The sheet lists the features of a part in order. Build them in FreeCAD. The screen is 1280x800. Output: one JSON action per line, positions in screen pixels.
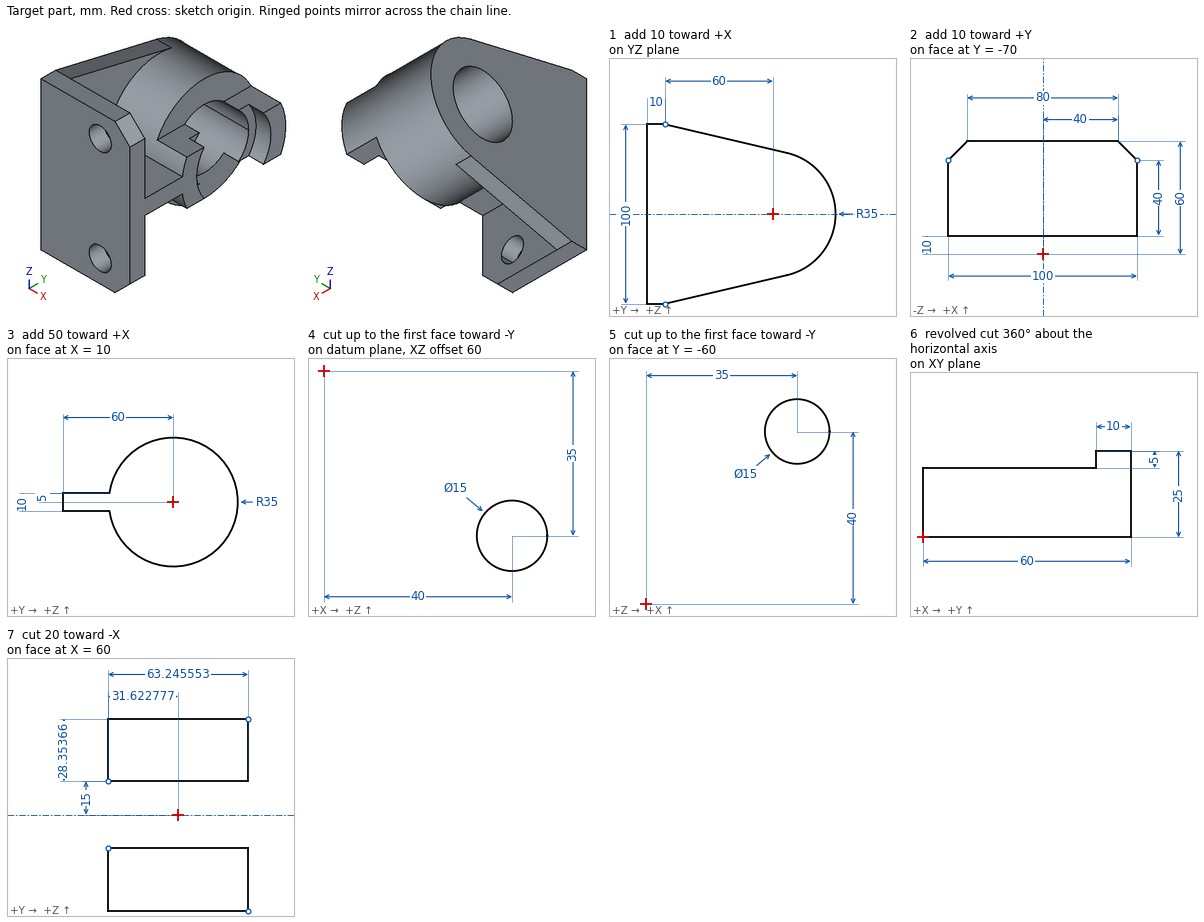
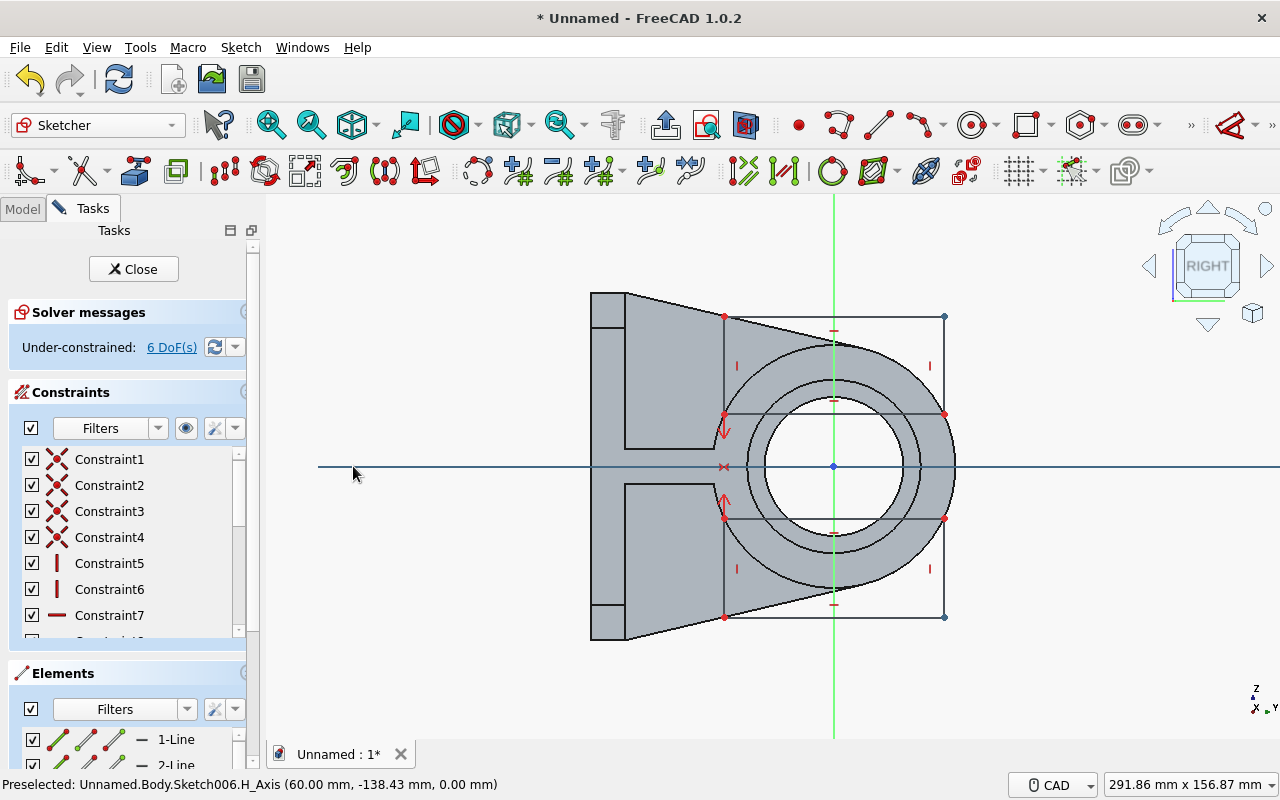
{"action": "key", "text": "s"}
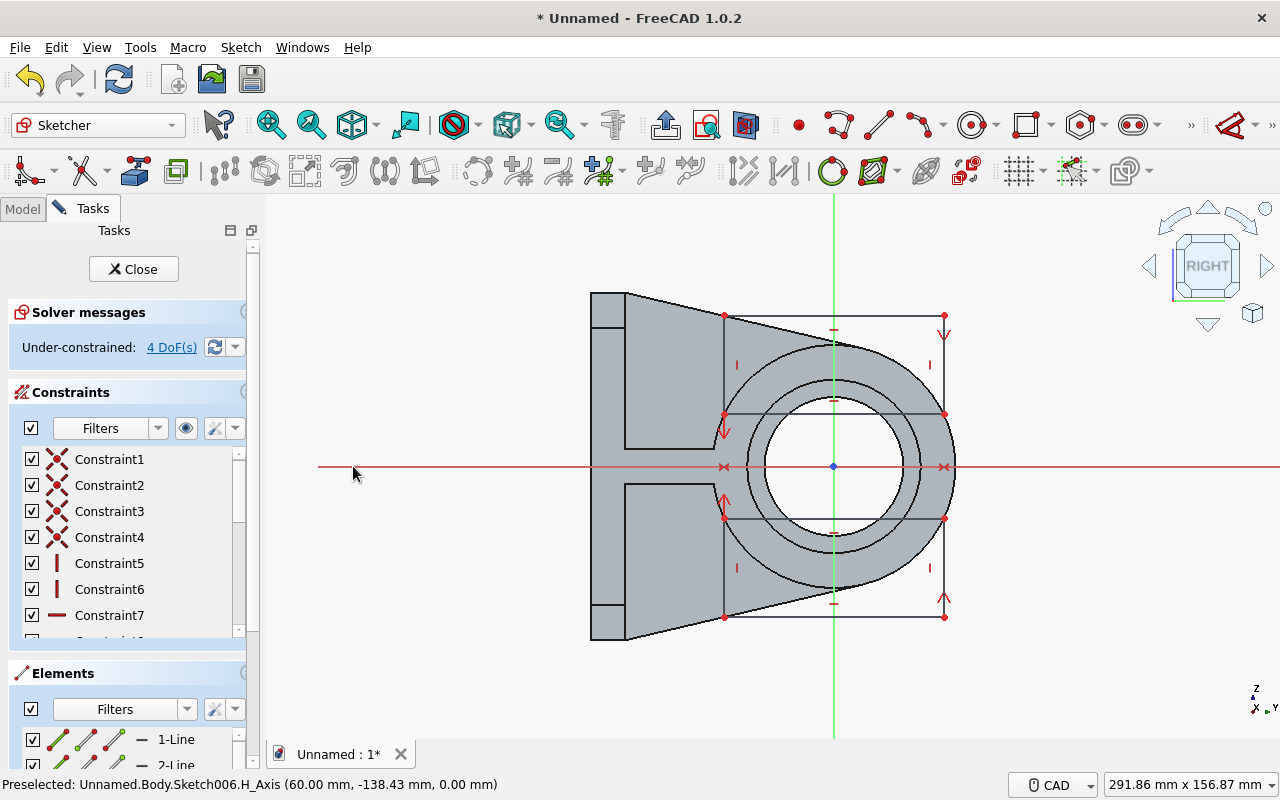
{"action": "left_click", "coordinate": [1230, 126]}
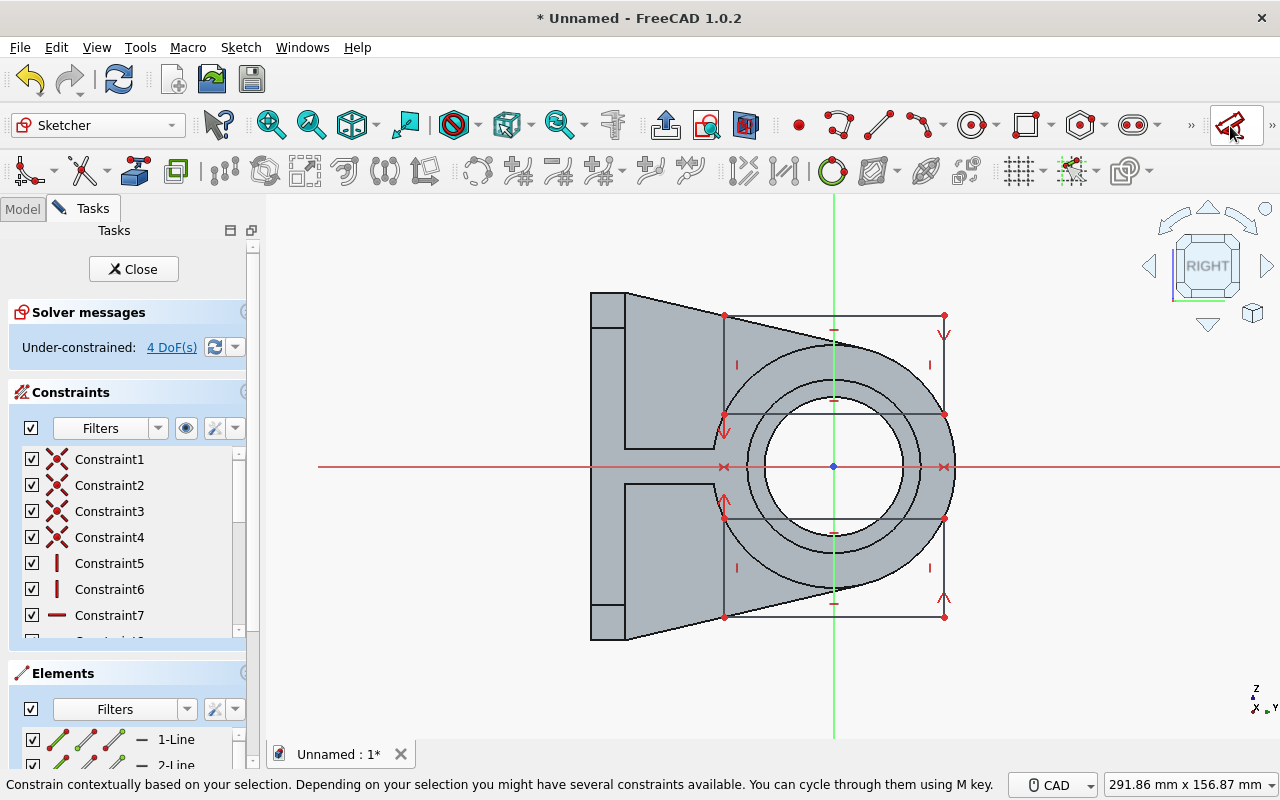
{"action": "left_click", "coordinate": [724, 414]}
{"action": "left_click", "coordinate": [690, 440]}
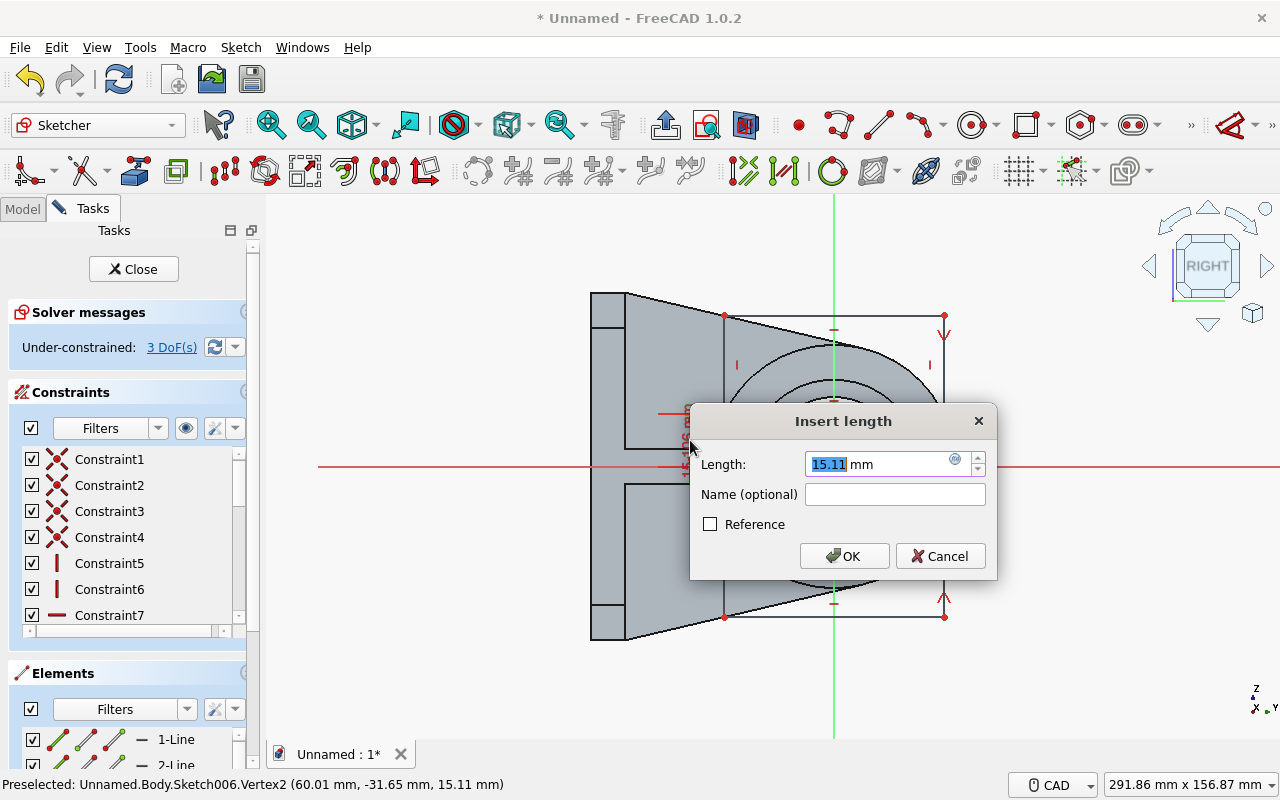
{"action": "type", "text": "15"}
{"action": "key", "text": "Return"}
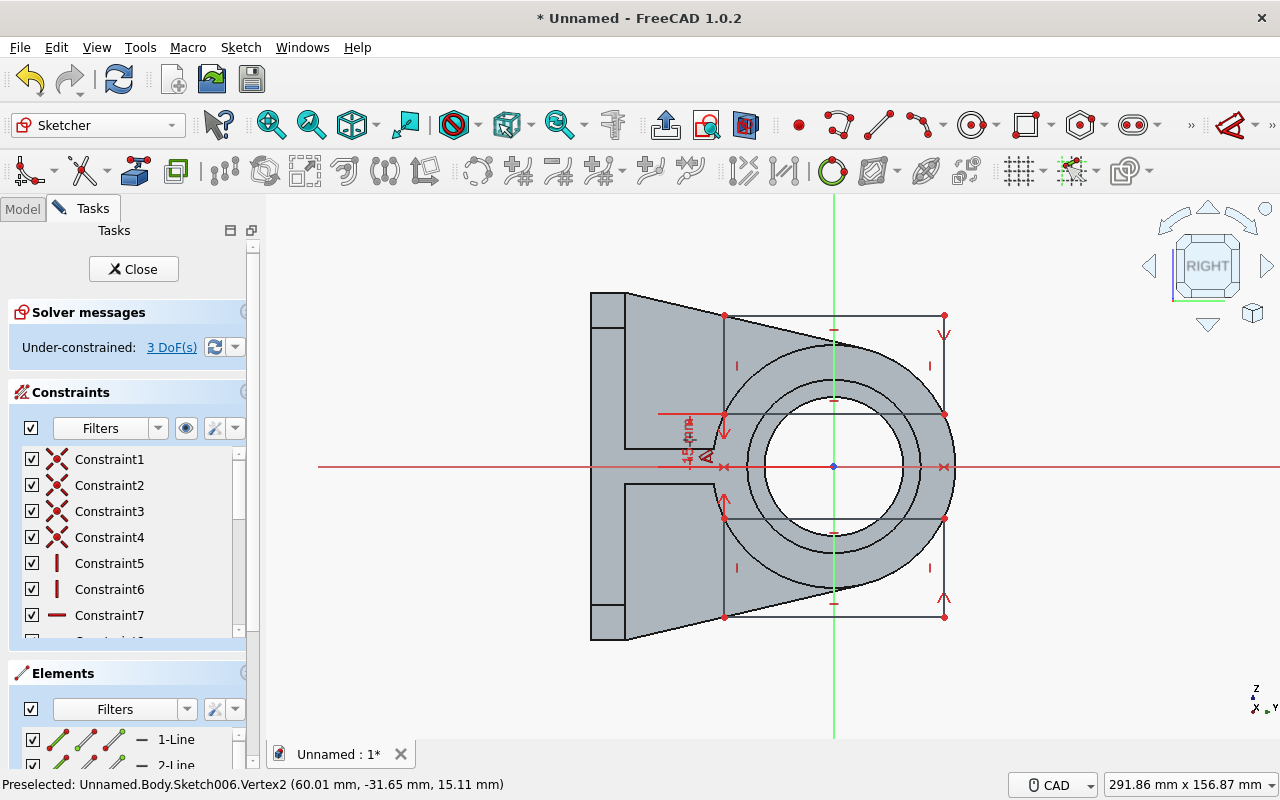
{"action": "left_click", "coordinate": [724, 346]}
{"action": "left_click", "coordinate": [690, 365]}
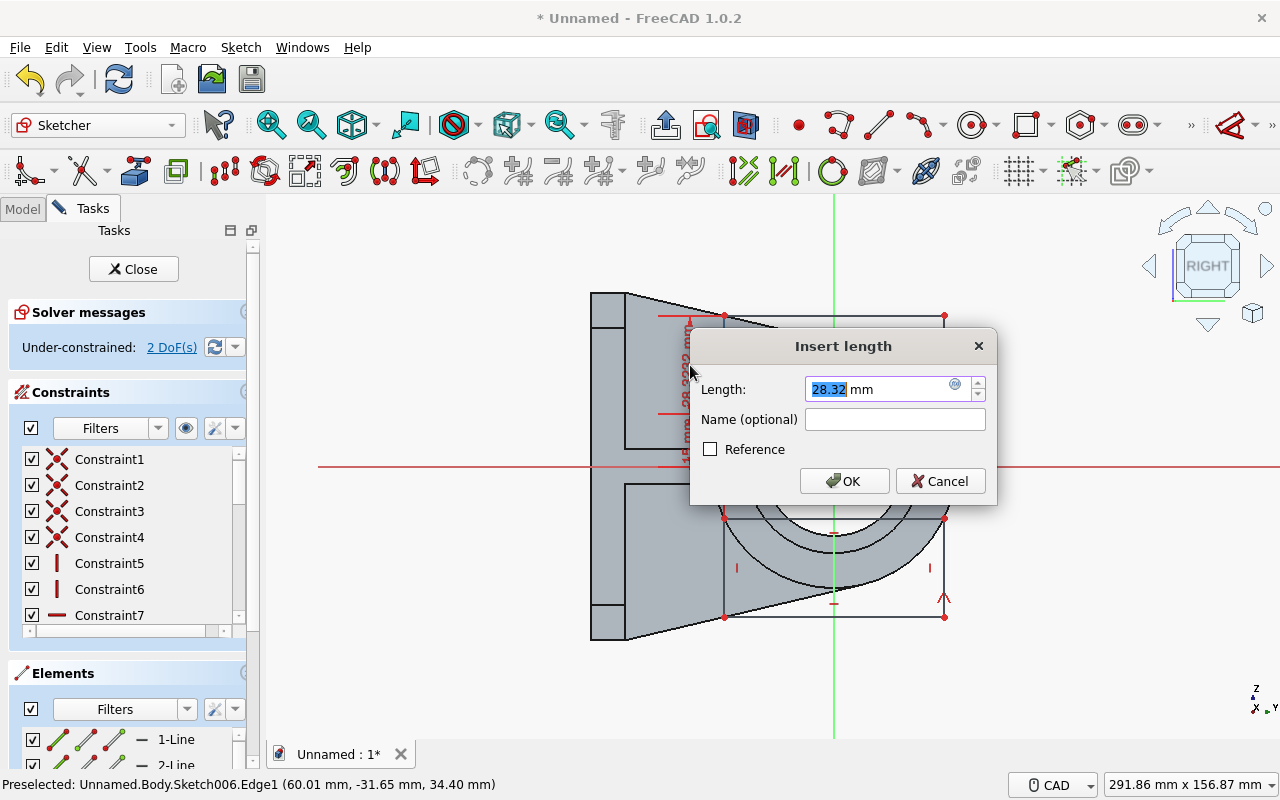
{"action": "type", "text": "28.35366"}
{"action": "key", "text": "Return"}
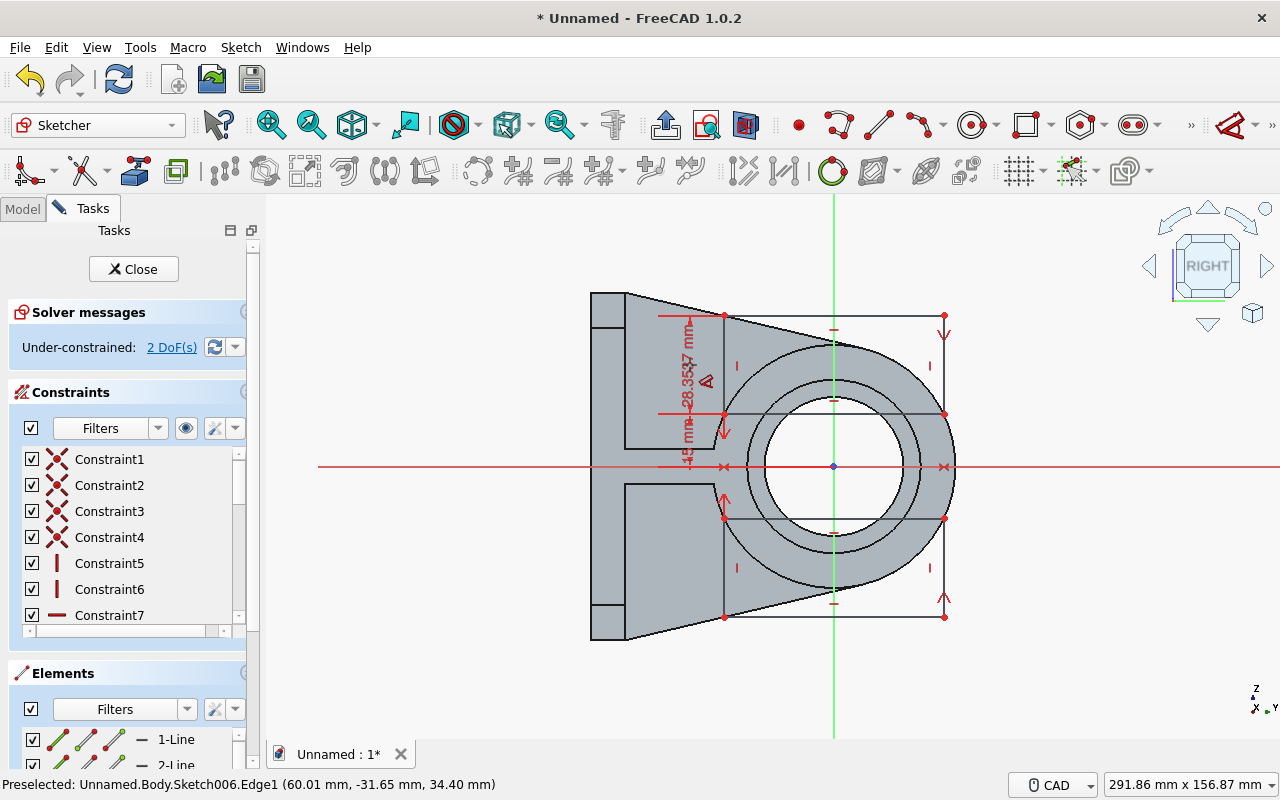
{"action": "left_click", "coordinate": [790, 414]}
{"action": "left_click", "coordinate": [783, 380]}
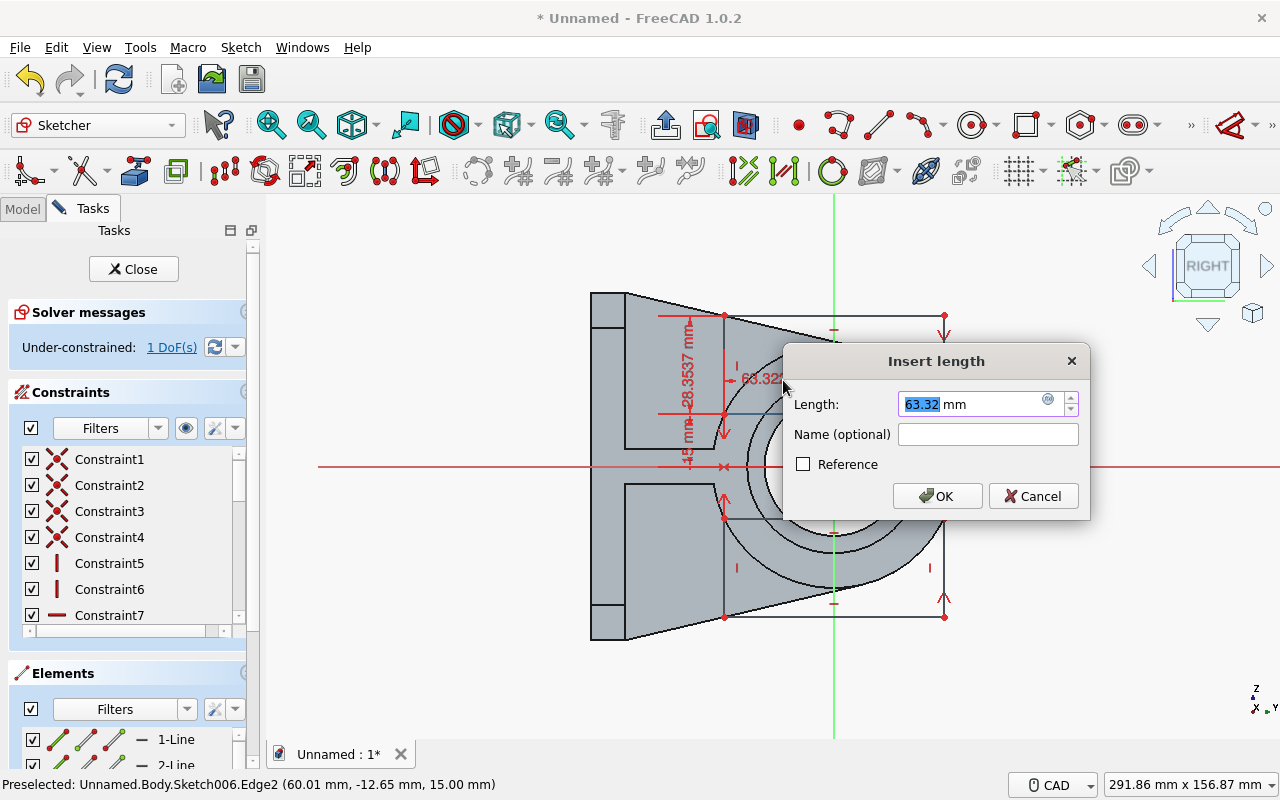
{"action": "type", "text": "63.245553"}
{"action": "key", "text": "Return"}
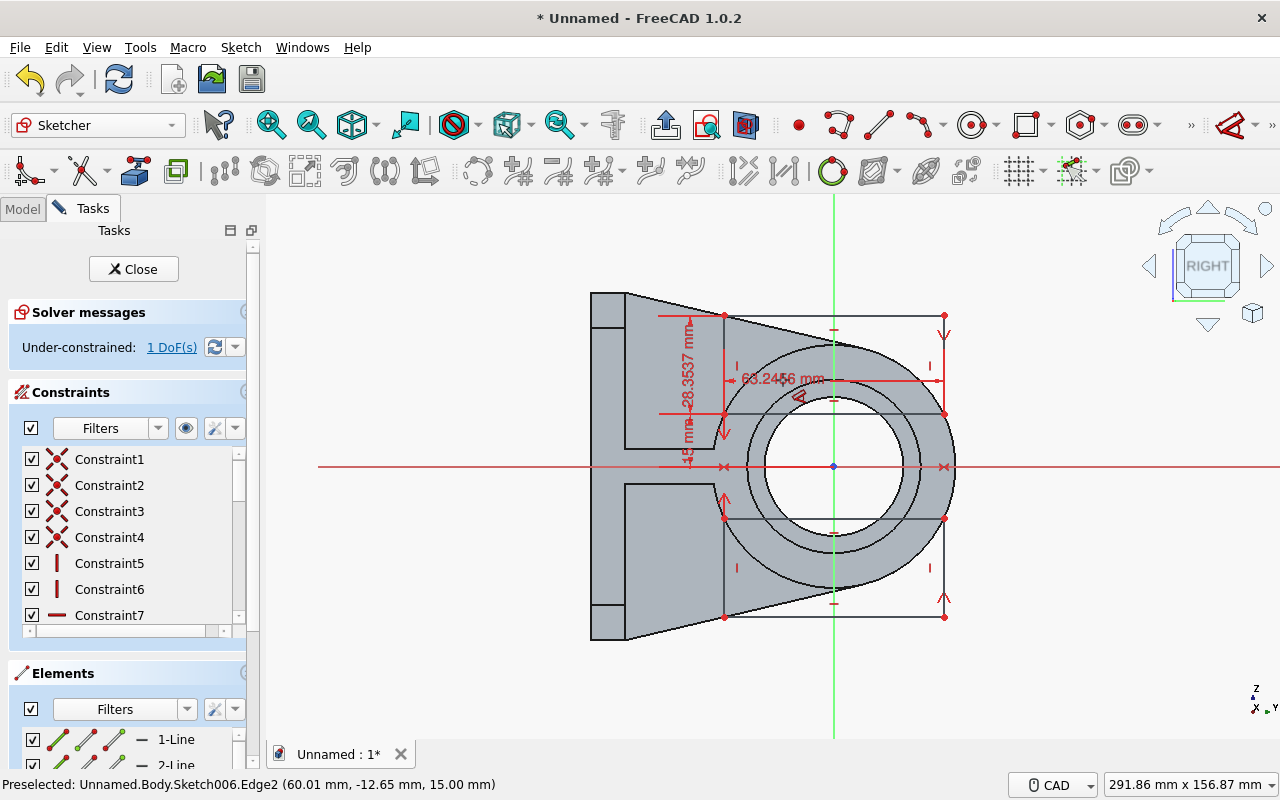
{"action": "left_click", "coordinate": [724, 316]}
{"action": "left_click", "coordinate": [779, 282]}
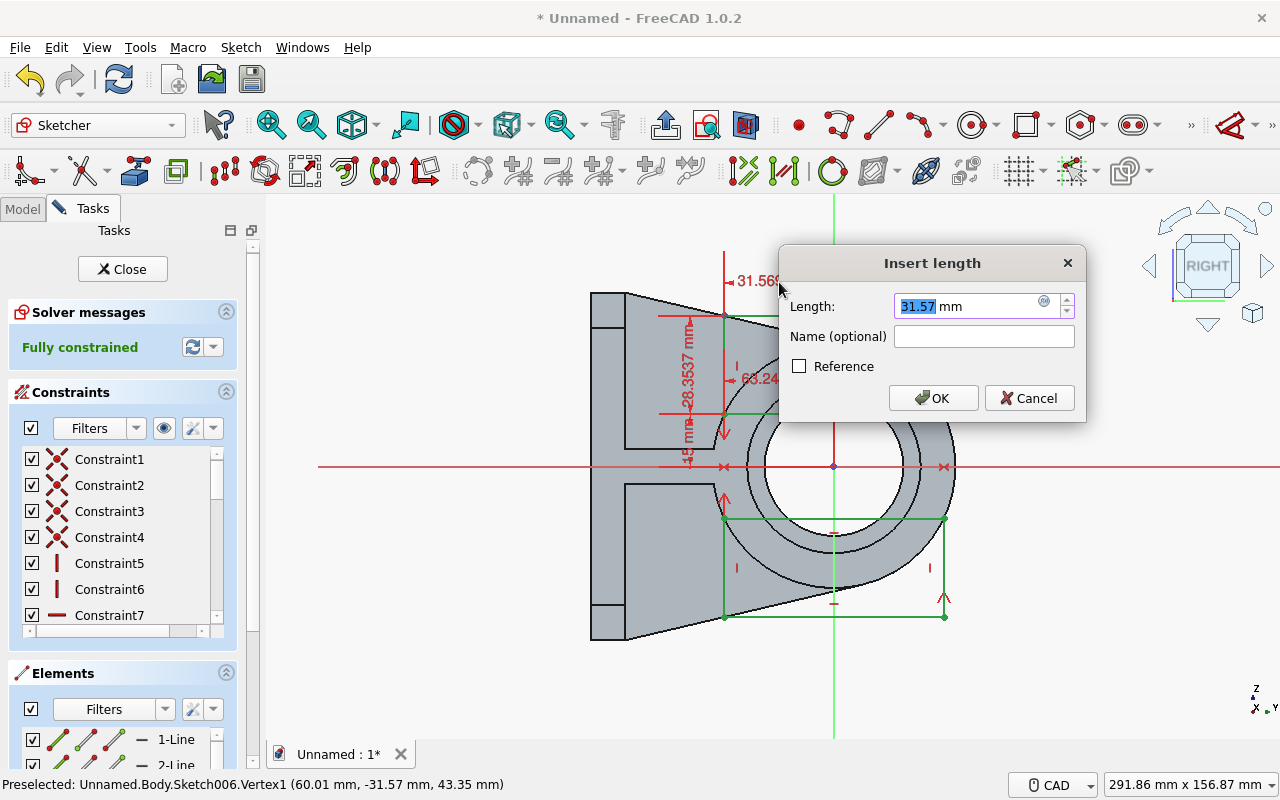
{"action": "type", "text": "31.622777"}
{"action": "key", "text": "Return"}
{"action": "key", "text": "Escape"}